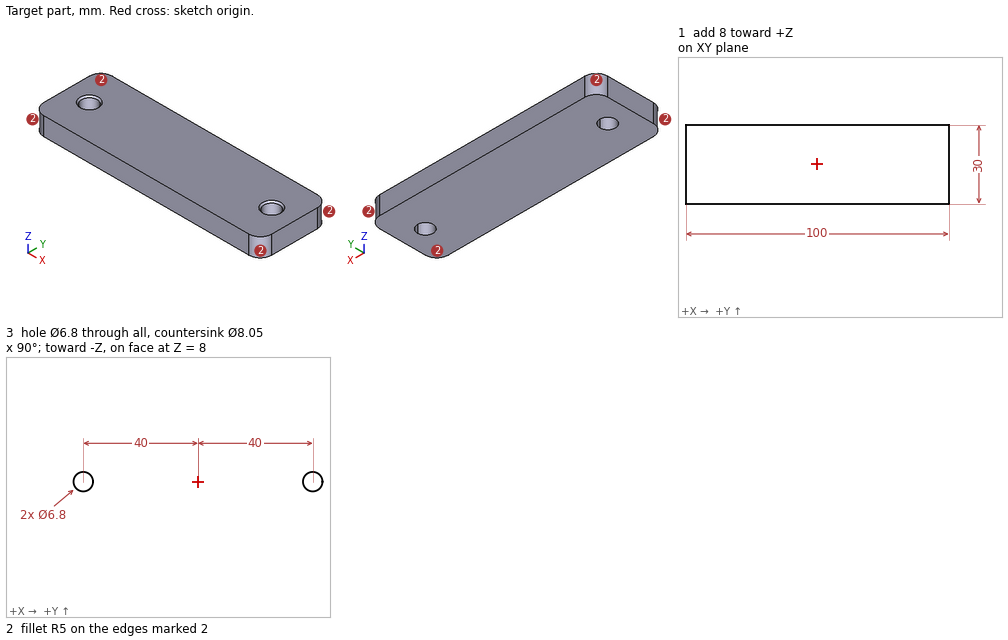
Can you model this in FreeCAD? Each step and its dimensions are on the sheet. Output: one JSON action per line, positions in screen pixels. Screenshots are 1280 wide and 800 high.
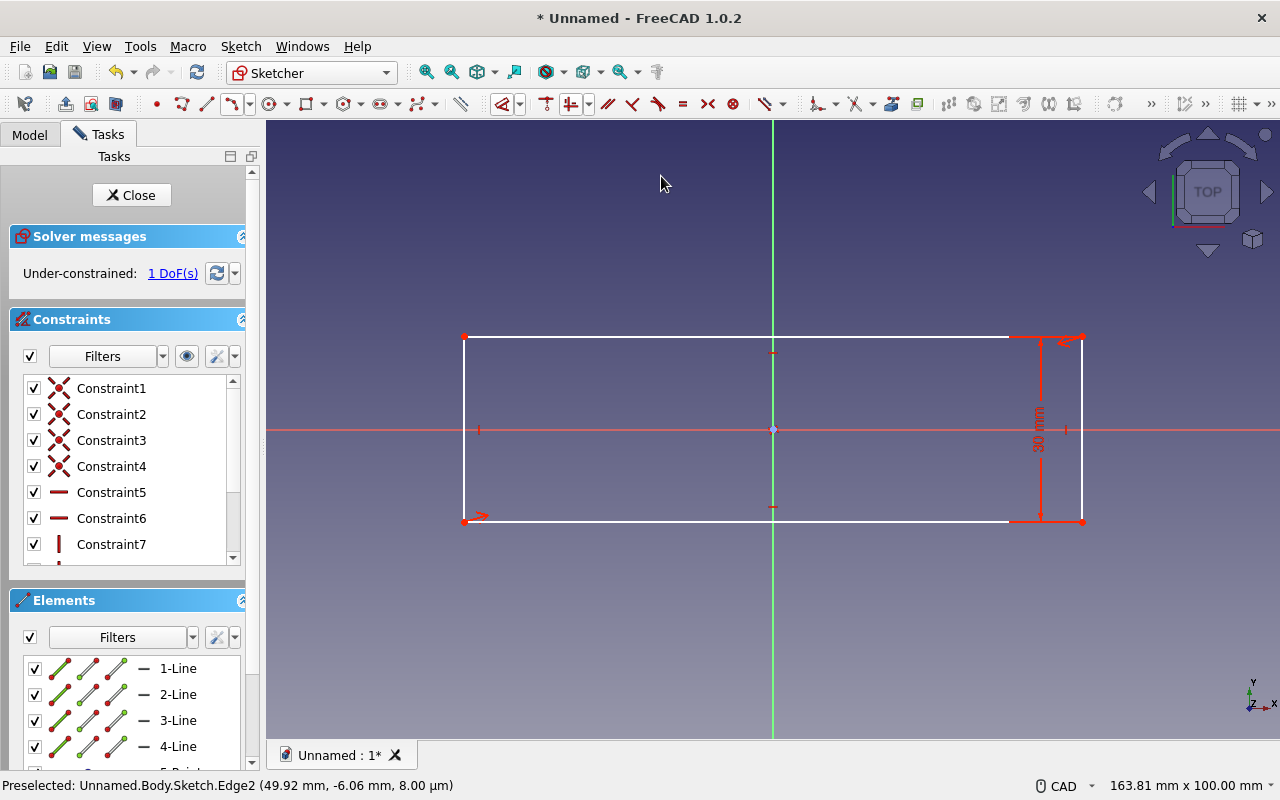
{"action": "left_click", "coordinate": [649, 522]}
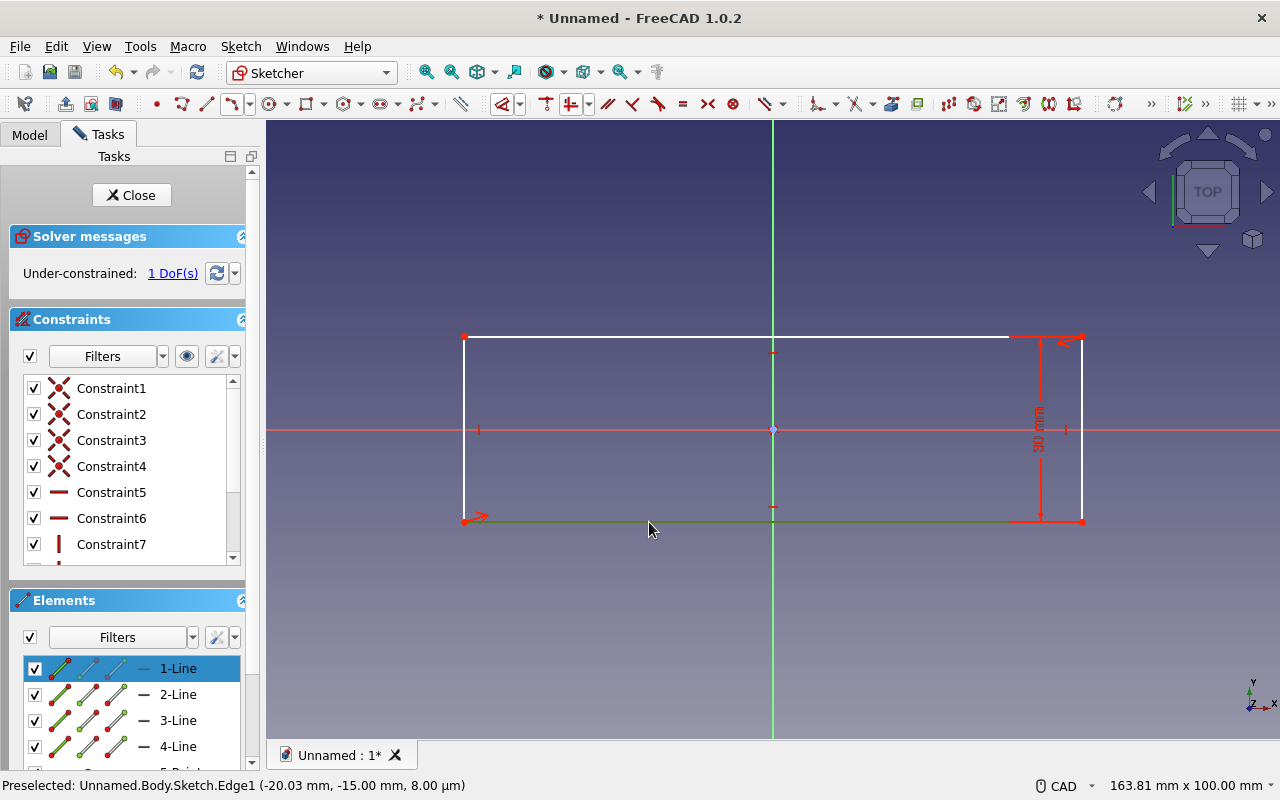
{"action": "key", "text": "l"}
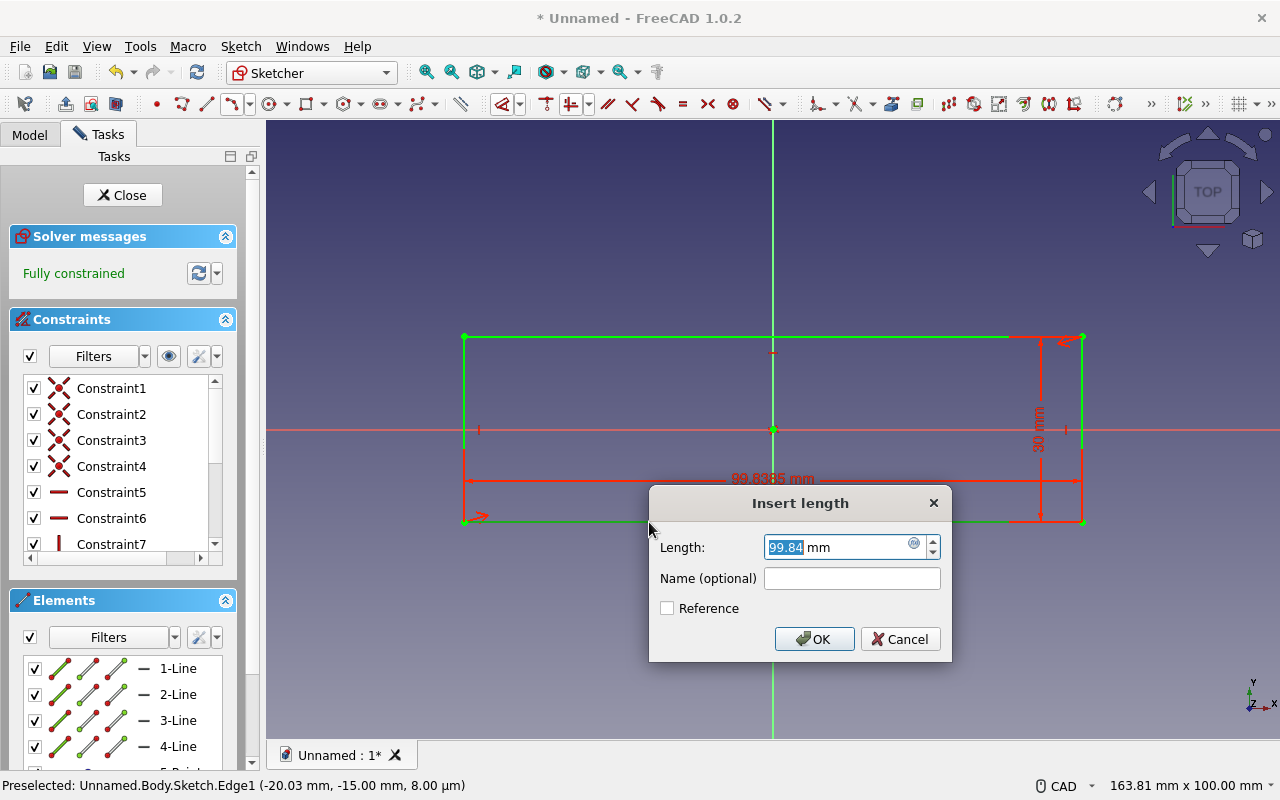
{"action": "type", "text": "100"}
{"action": "key", "text": "Return"}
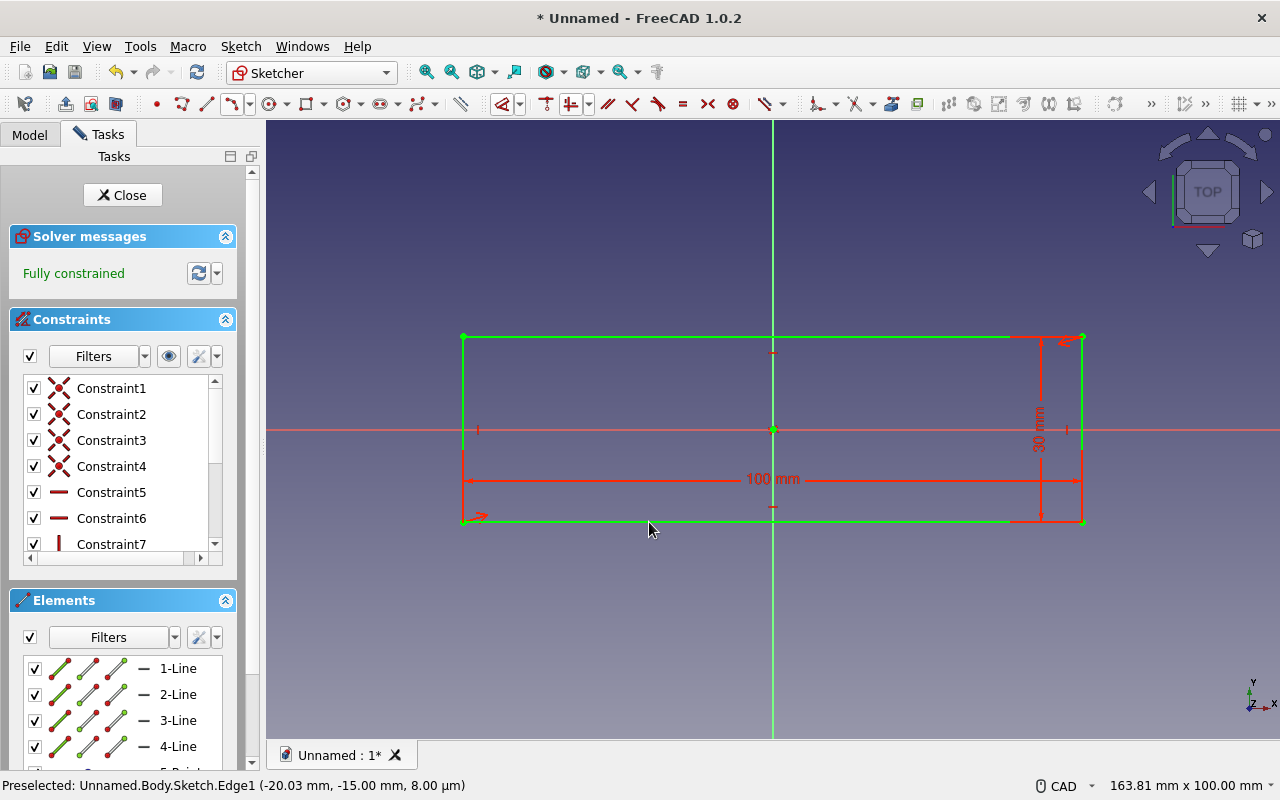
{"action": "left_click", "coordinate": [123, 195]}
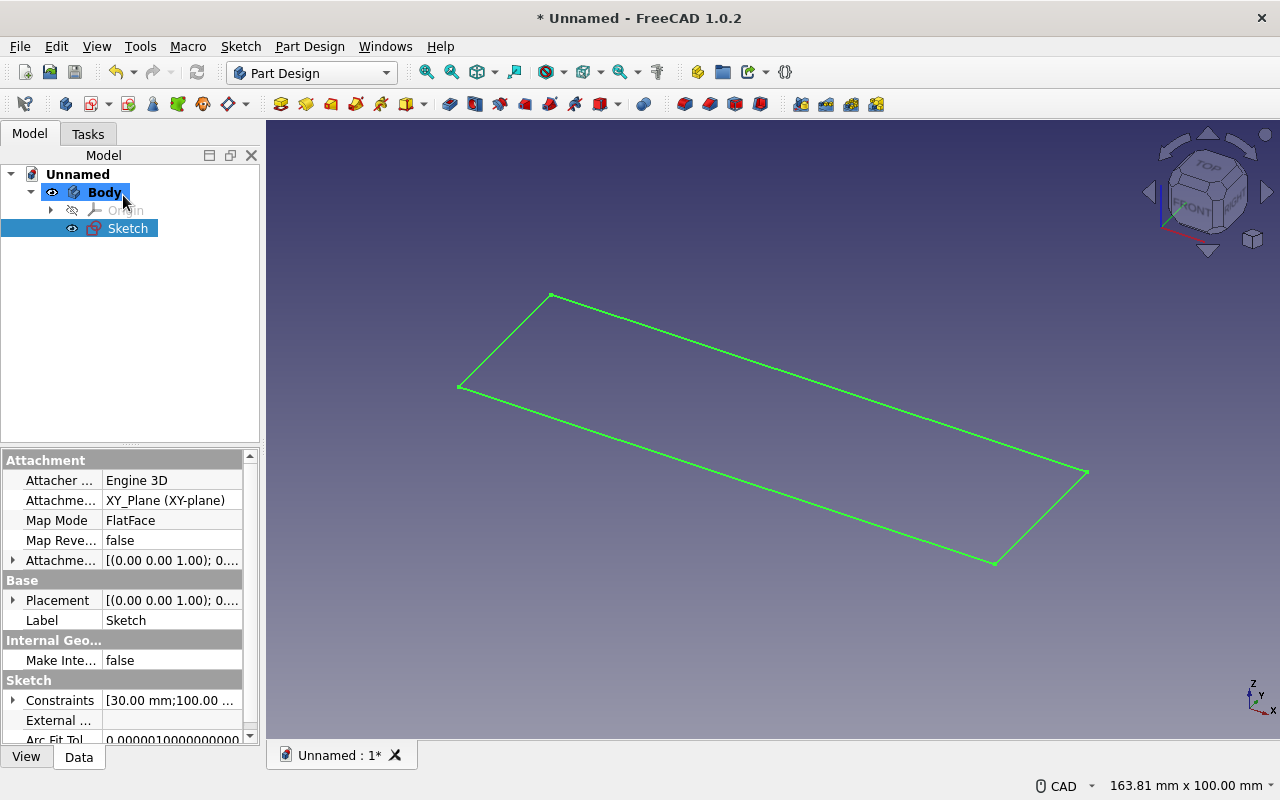
{"action": "left_click", "coordinate": [281, 104]}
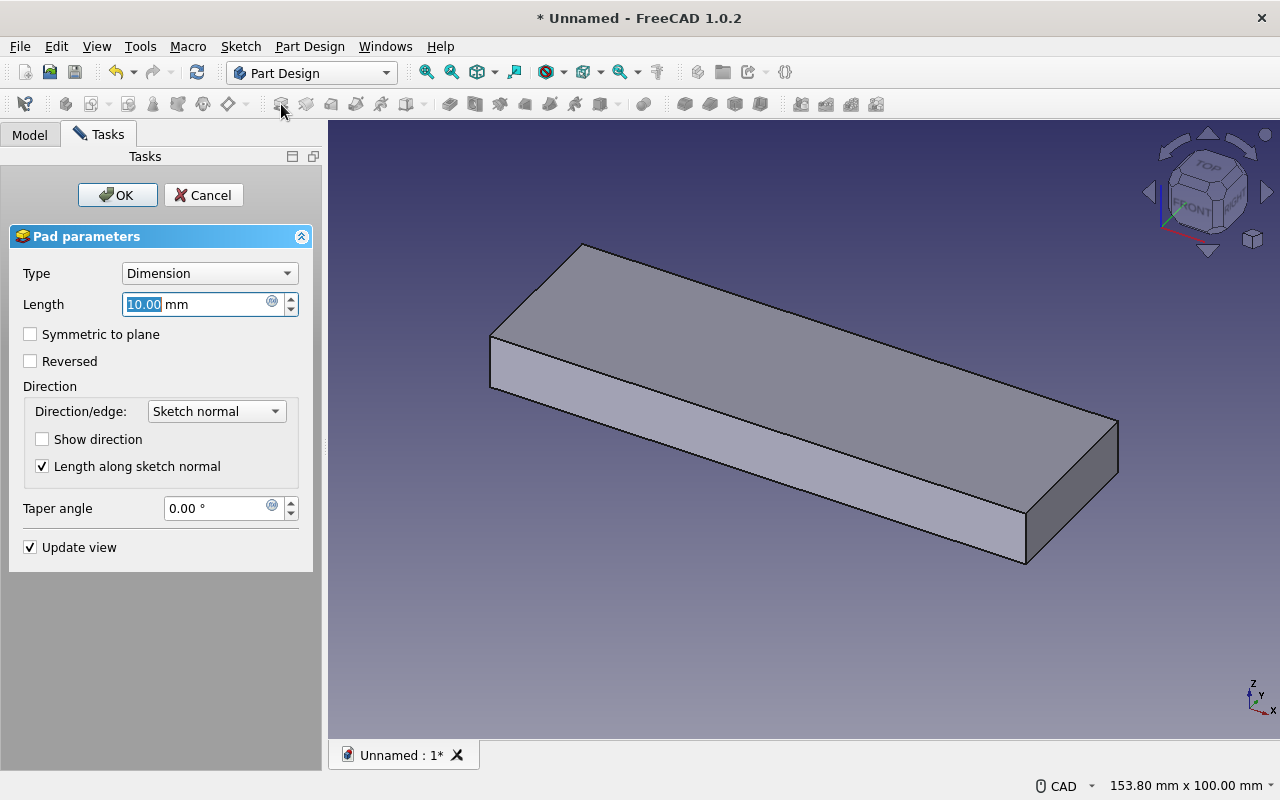
{"action": "type", "text": "8"}
{"action": "key", "text": "Tab"}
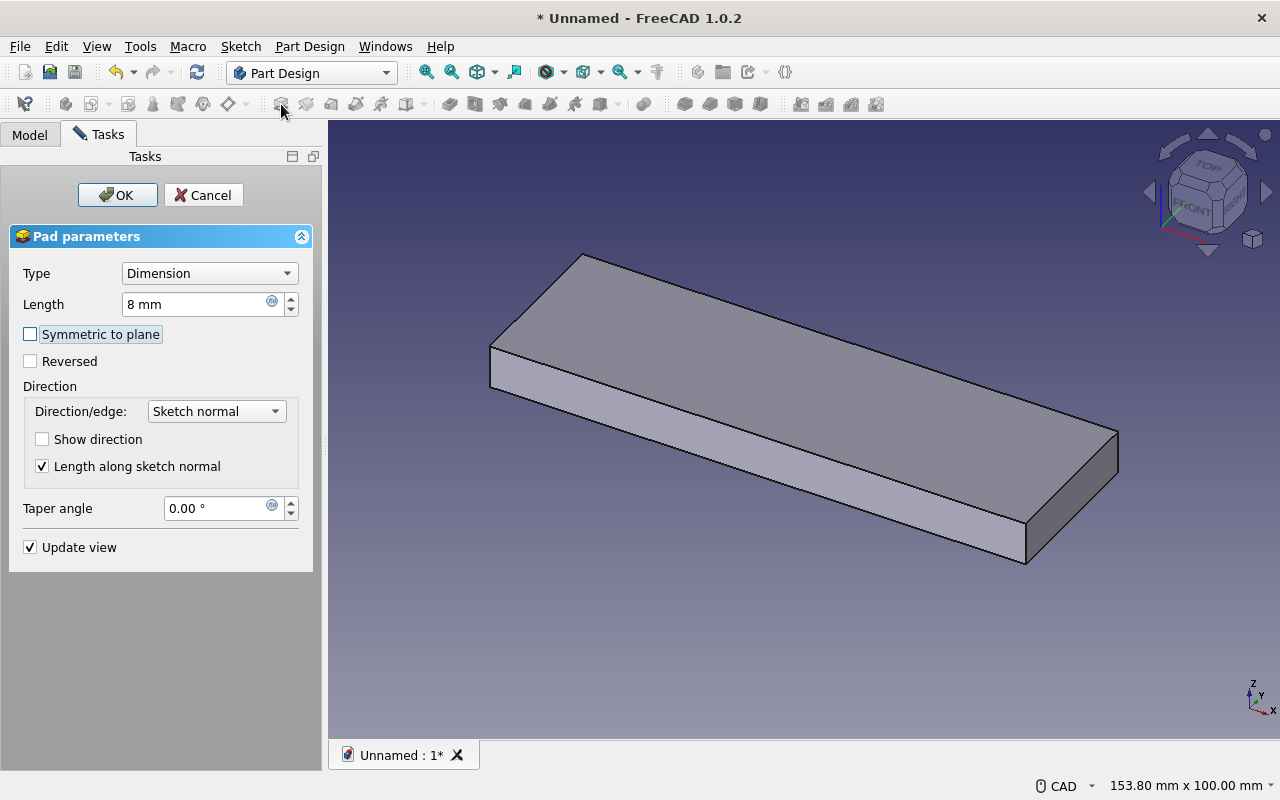
{"action": "left_click", "coordinate": [118, 195]}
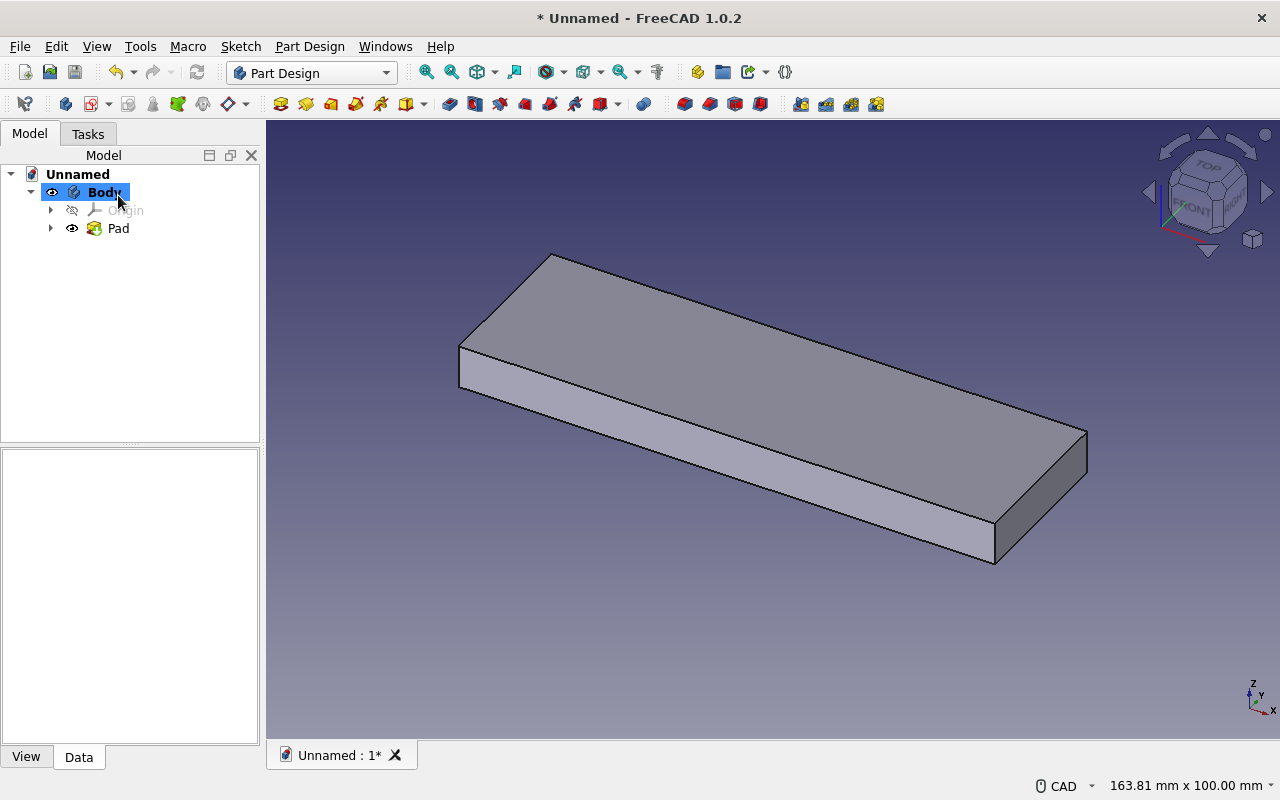
{"action": "left_click", "coordinate": [995, 543]}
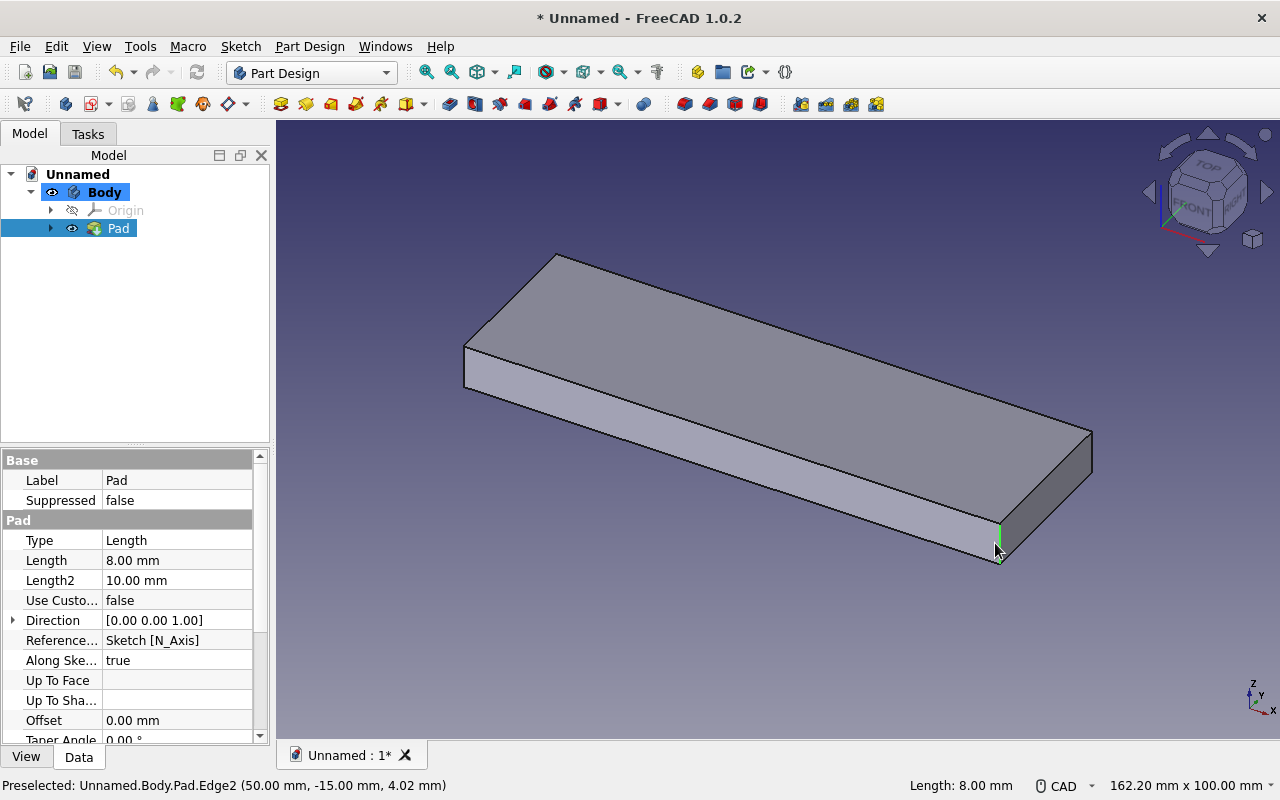
{"action": "key", "text": "0"}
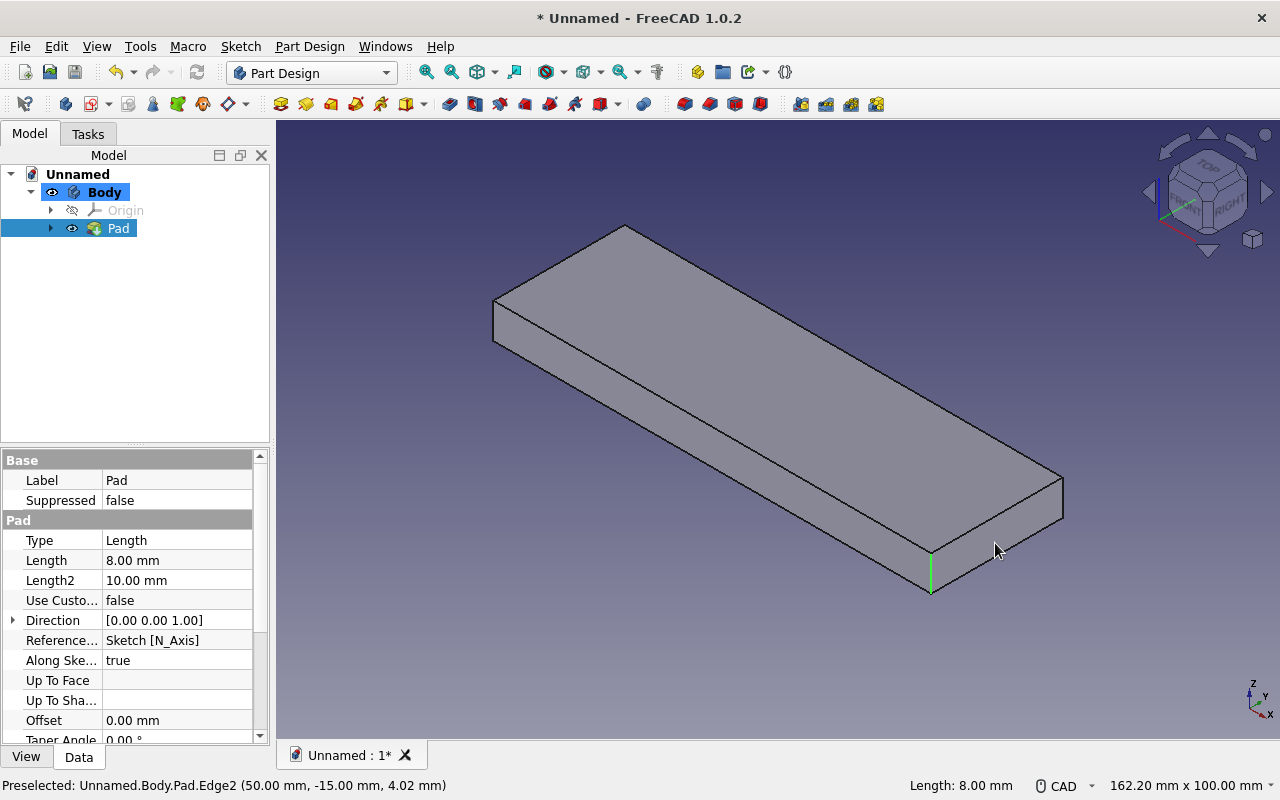
{"action": "key", "text": "2"}